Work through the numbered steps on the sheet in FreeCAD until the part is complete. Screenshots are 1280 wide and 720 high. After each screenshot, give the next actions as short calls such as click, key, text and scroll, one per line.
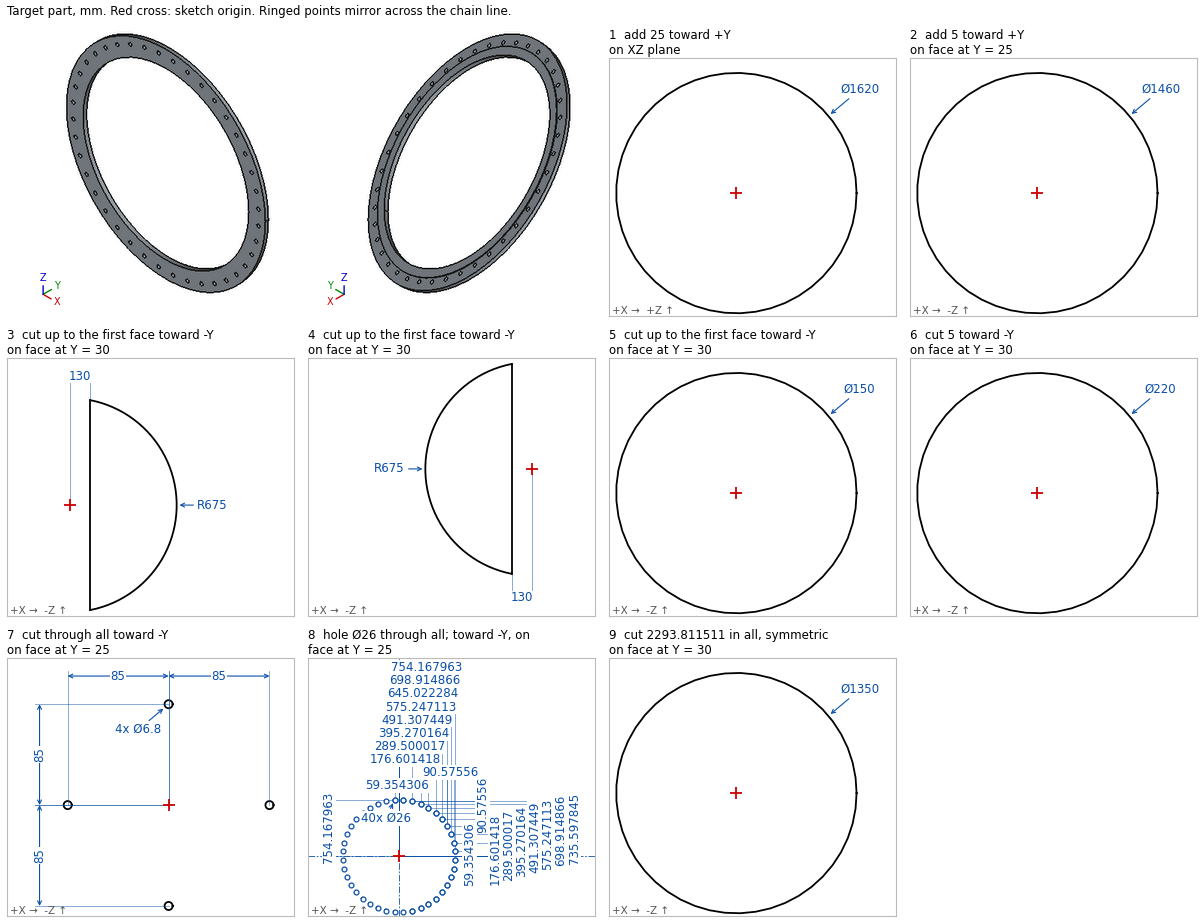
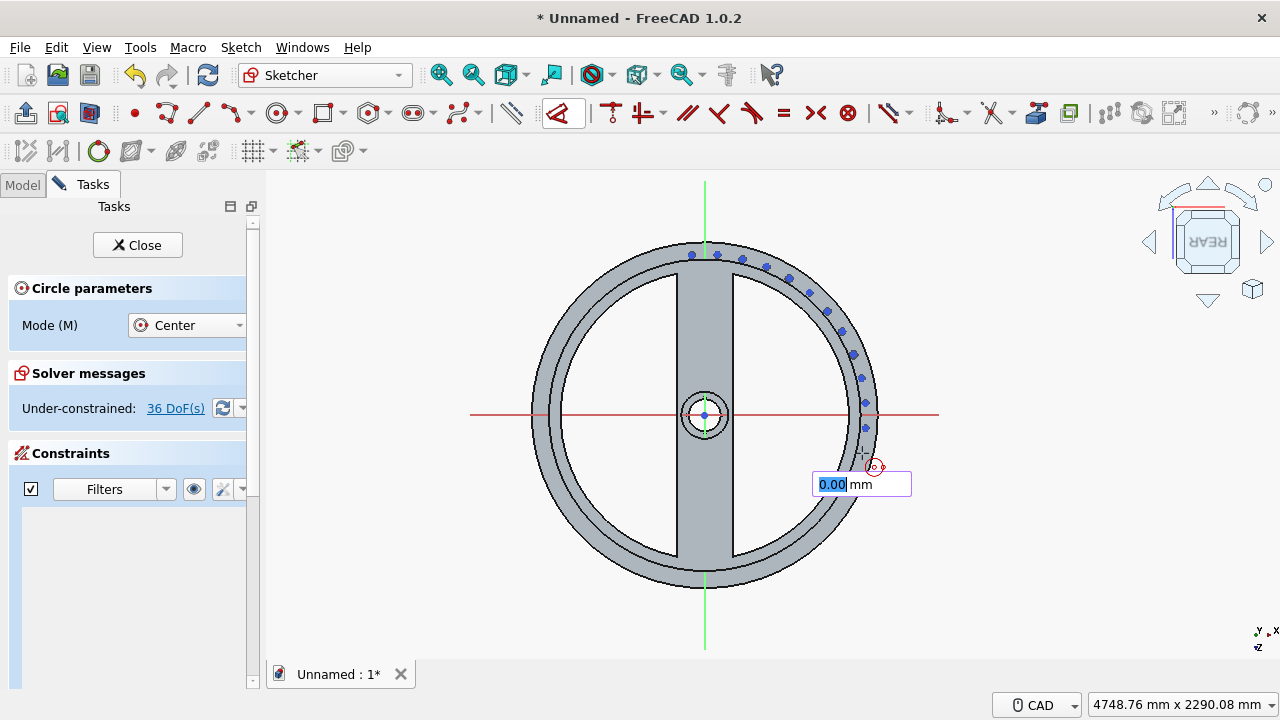
scroll(864, 451, up, 9)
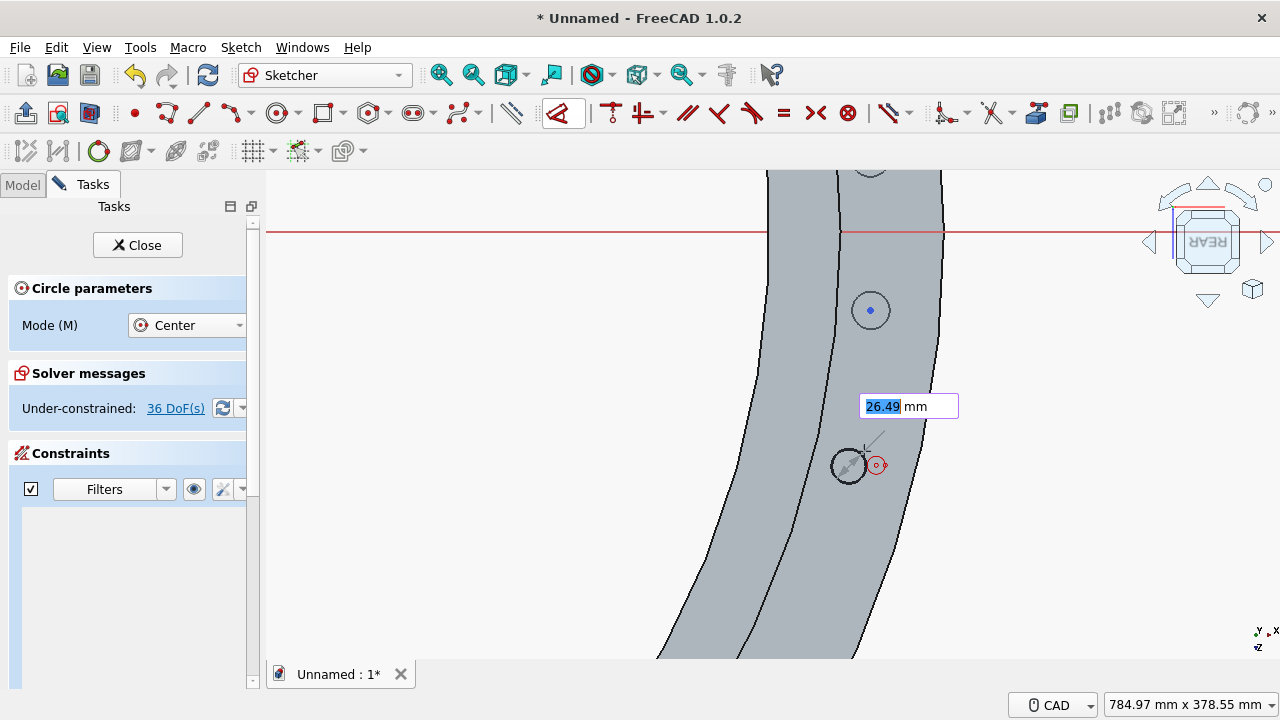
click(860, 448)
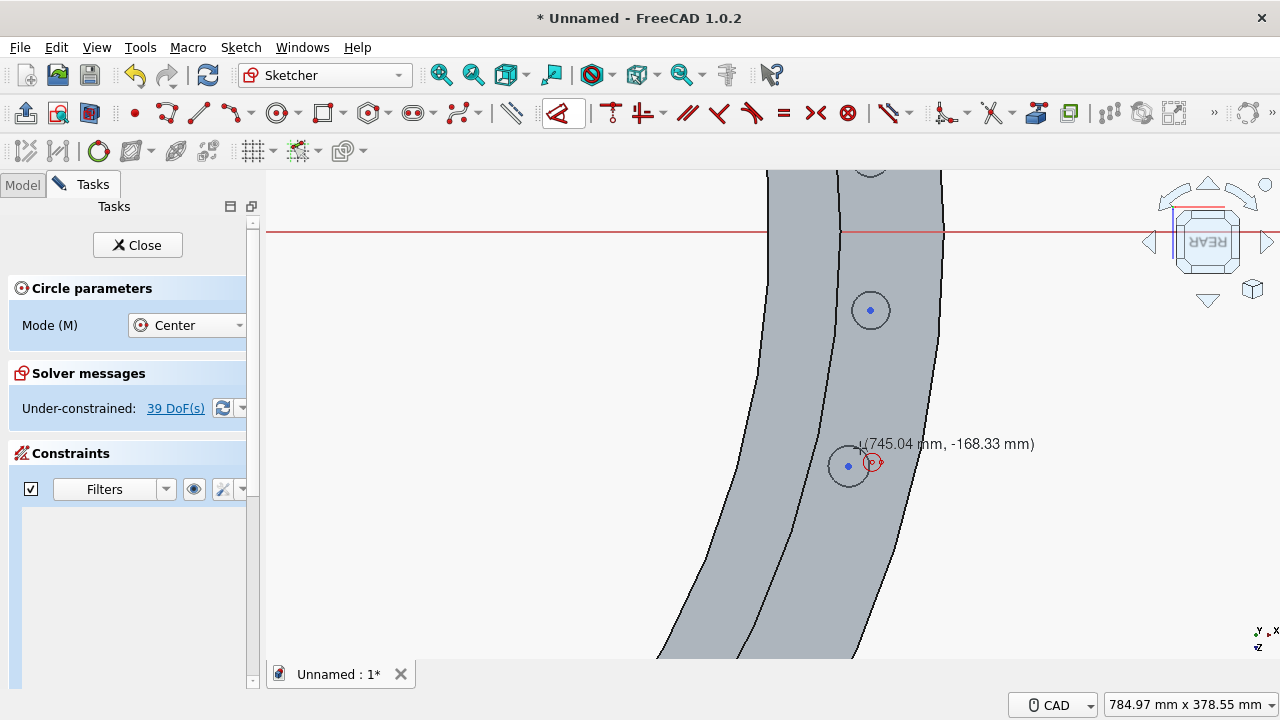
scroll(800, 606, up, 2)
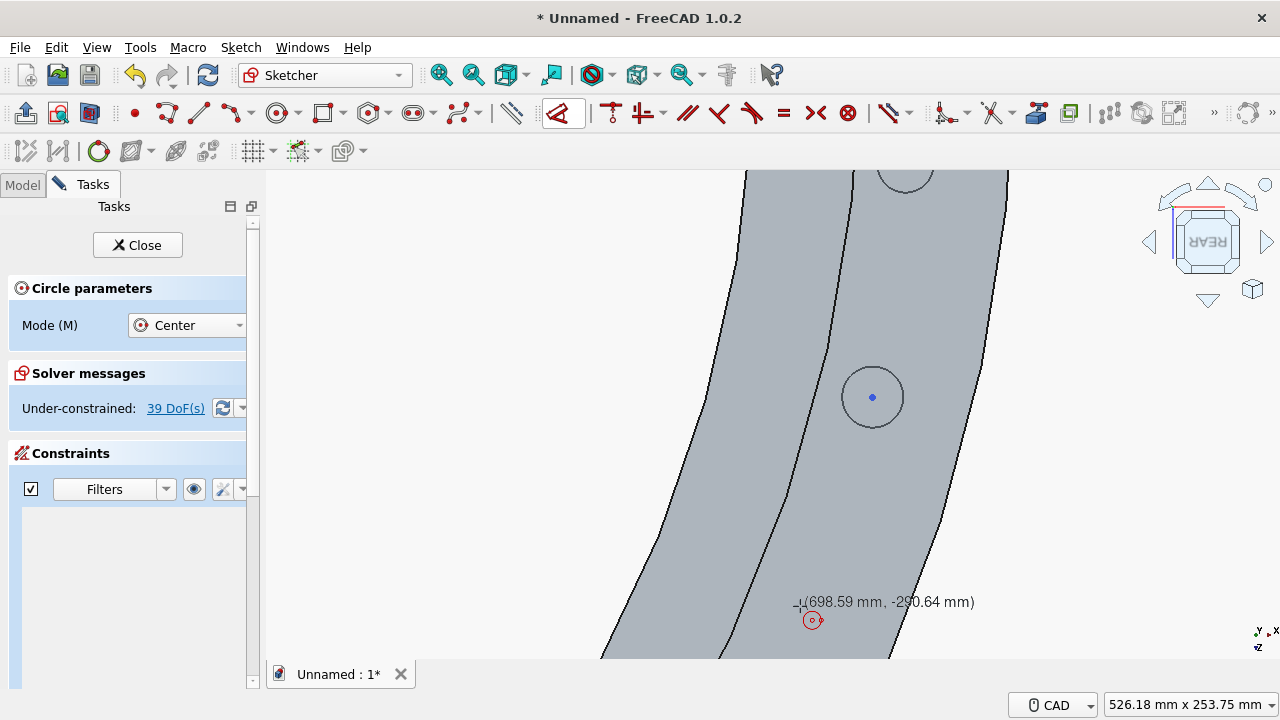
scroll(860, 460, down, 11)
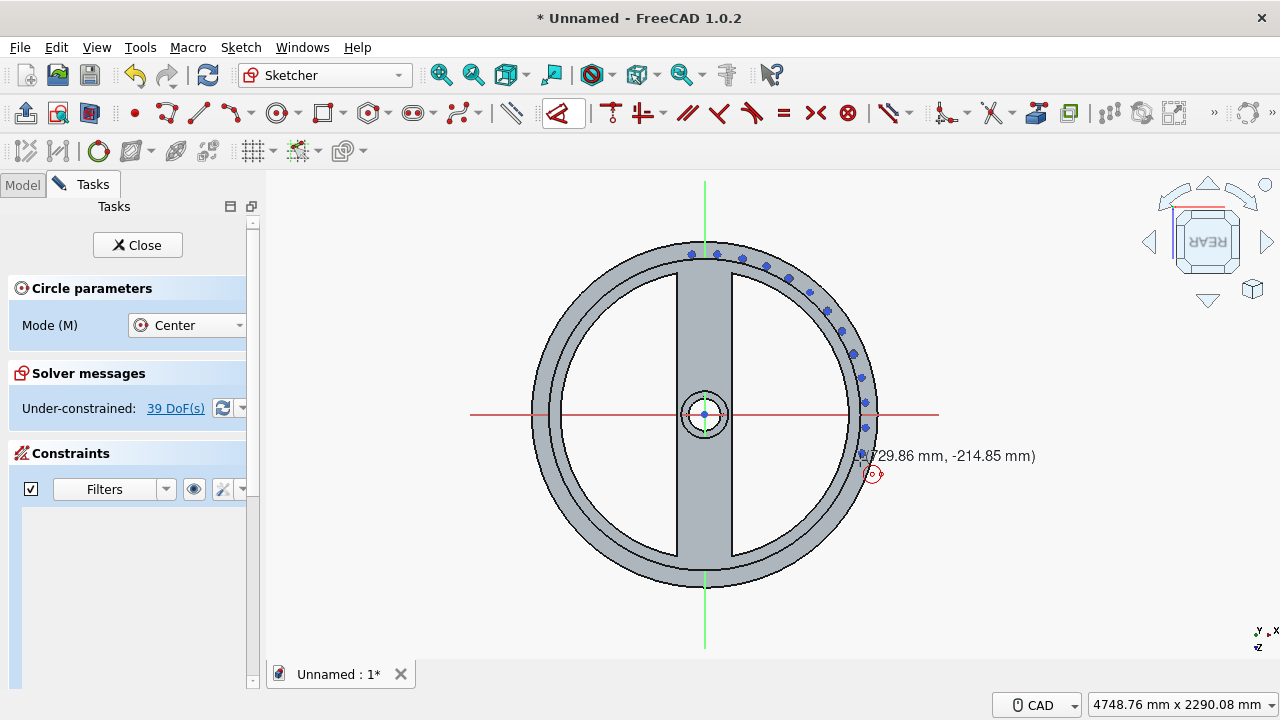
click(854, 477)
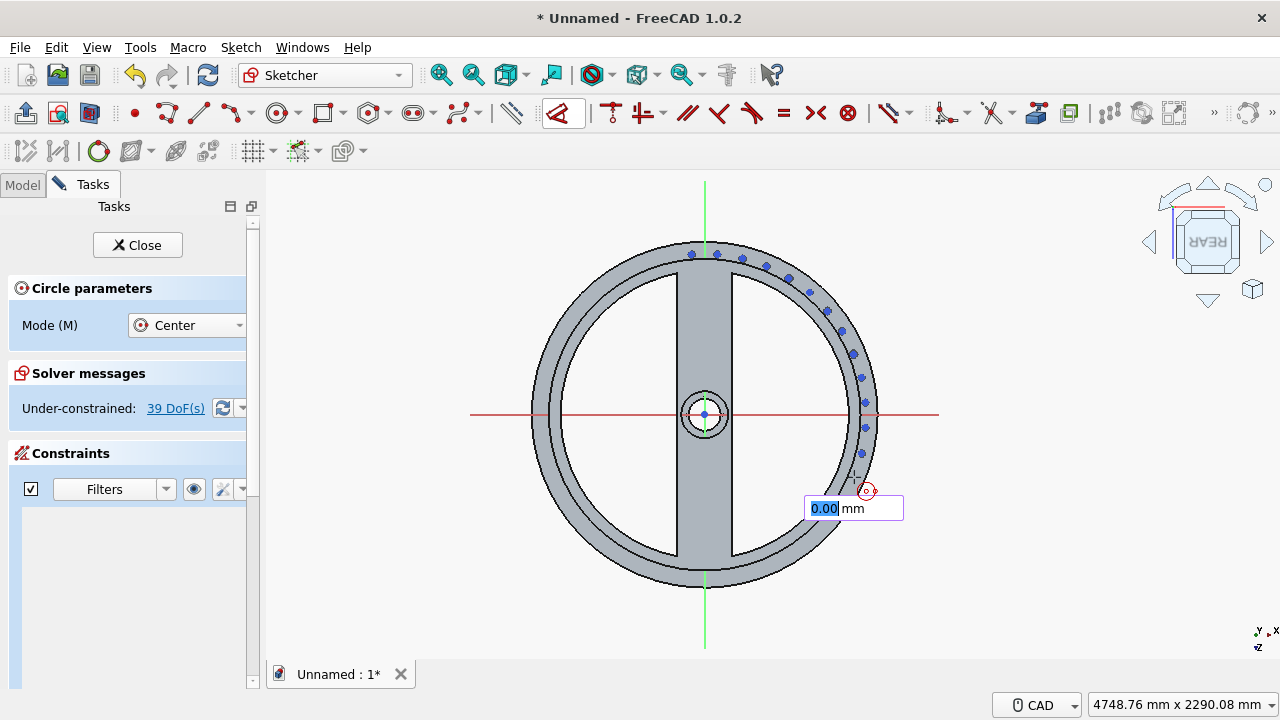
scroll(856, 475, up, 9)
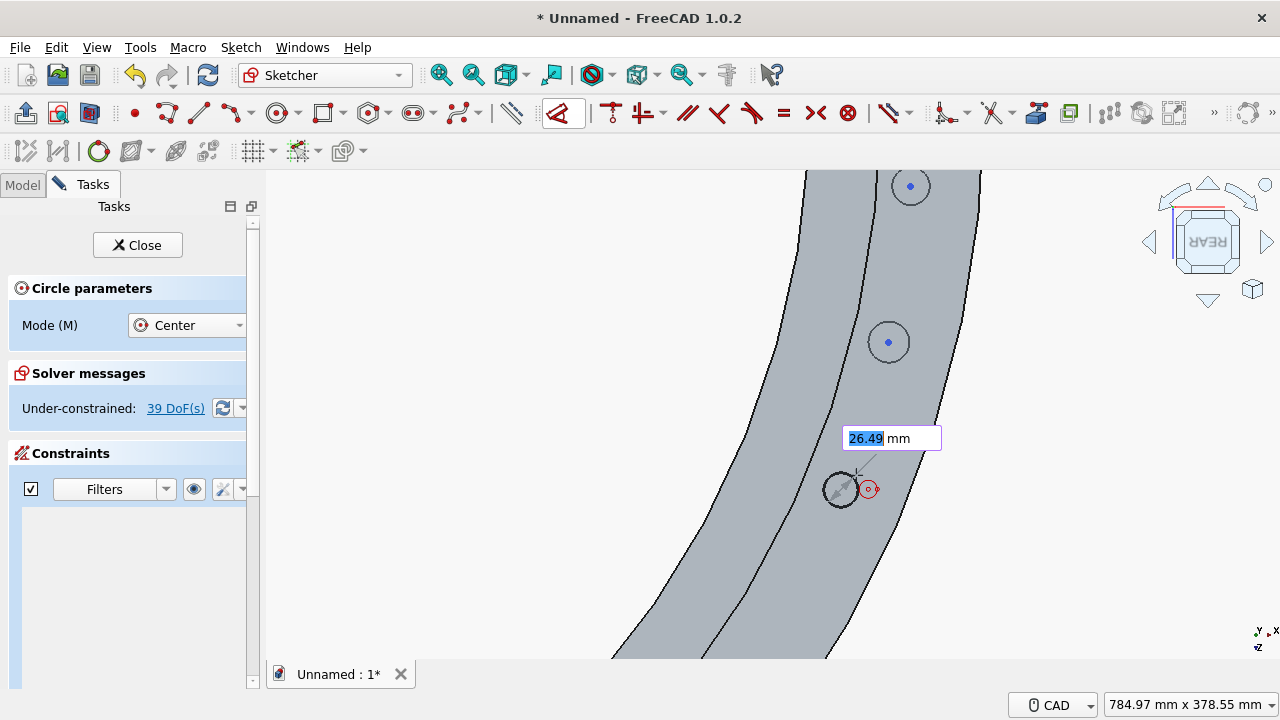
click(852, 470)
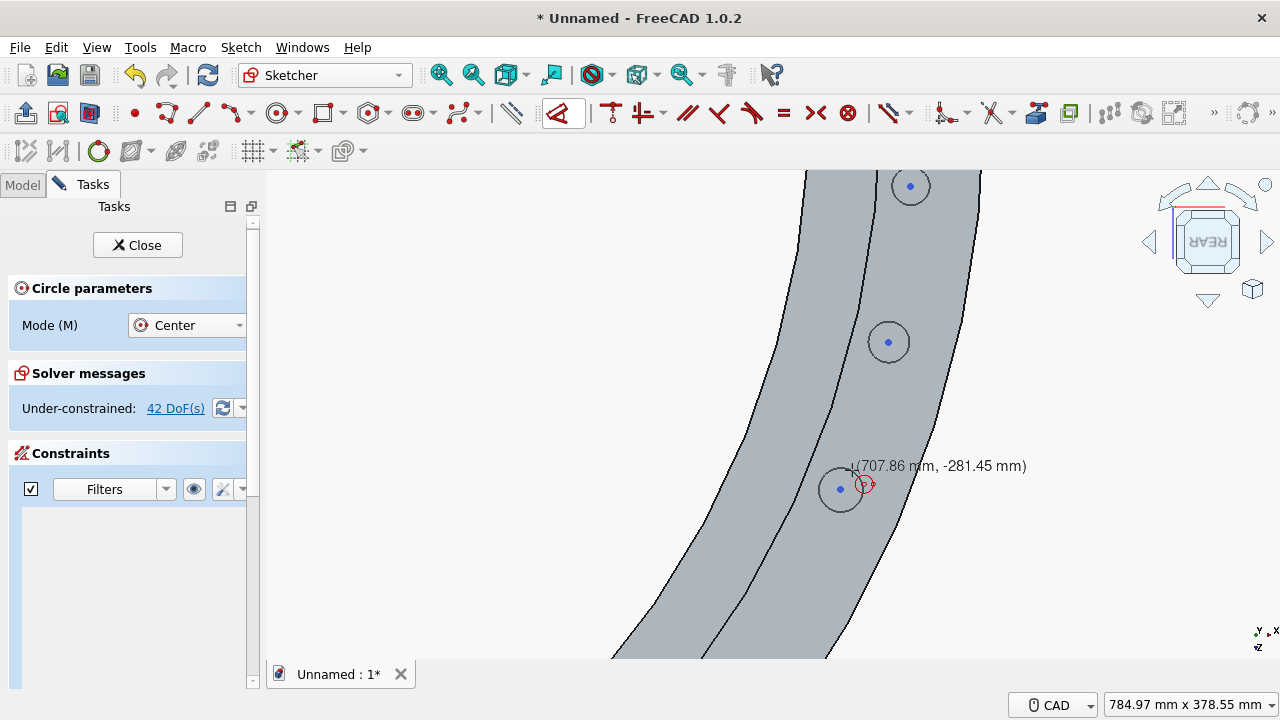
scroll(771, 618, up, 2)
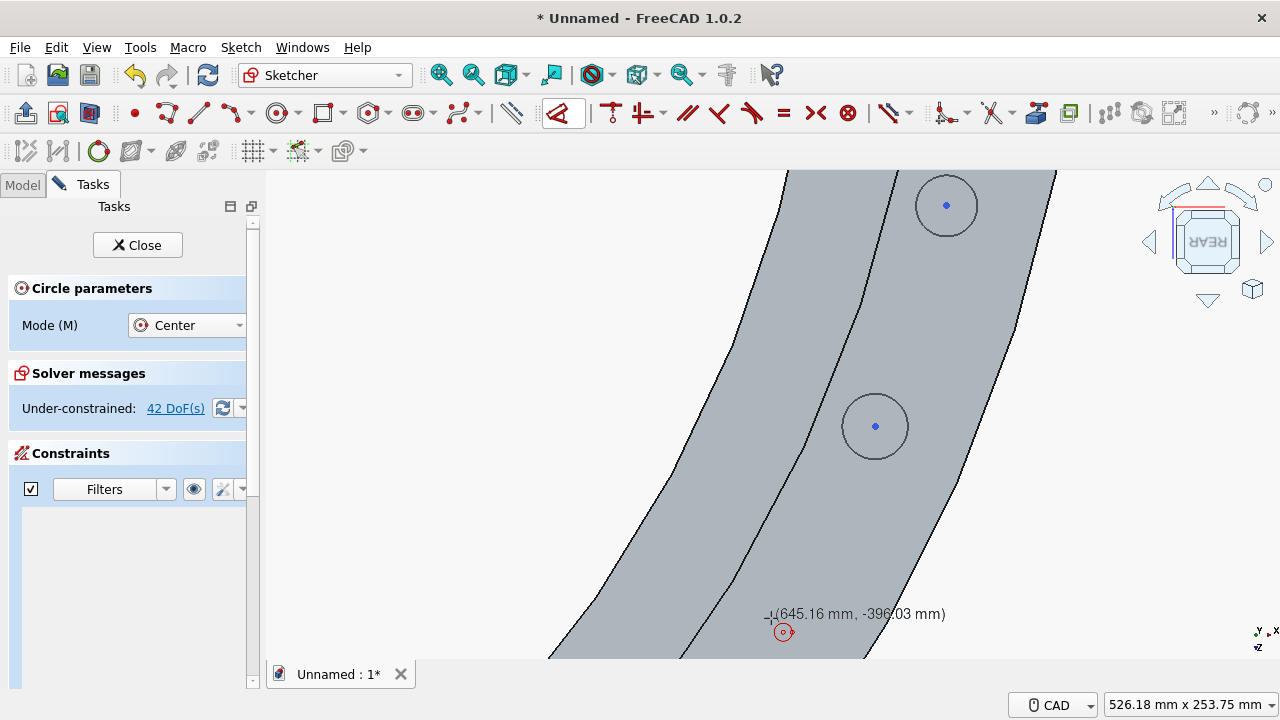
scroll(851, 484, down, 11)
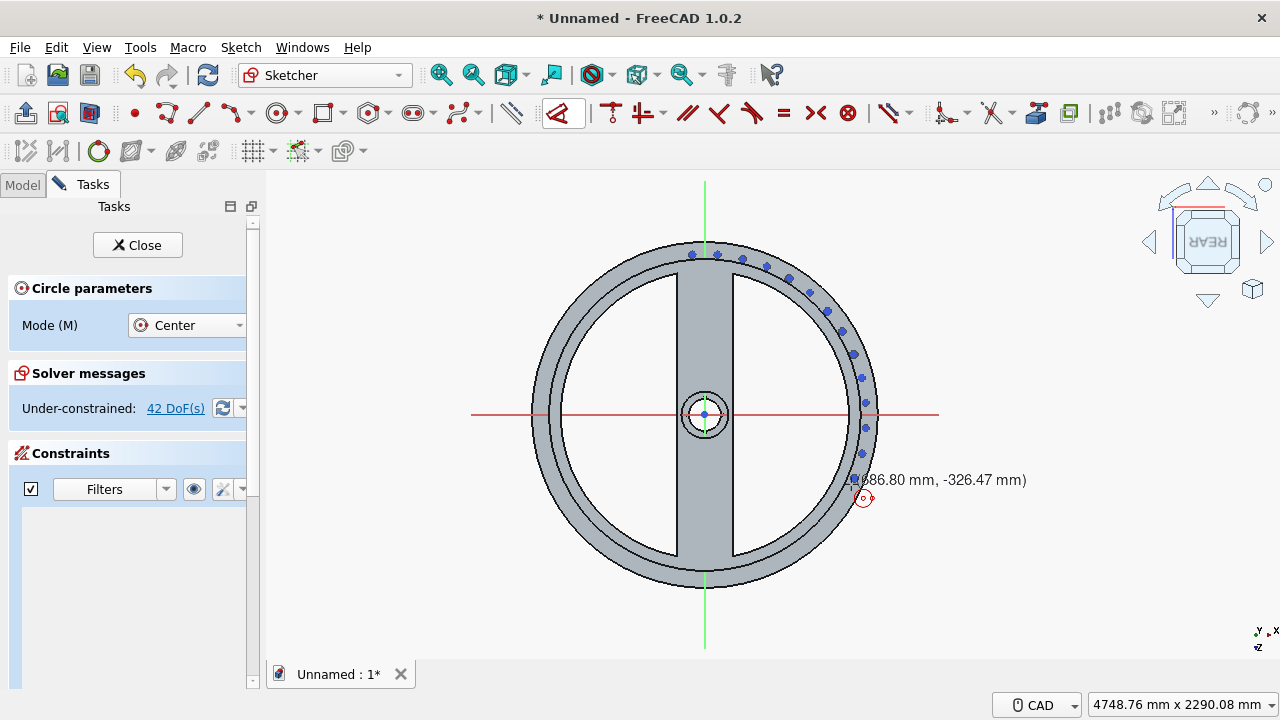
click(843, 499)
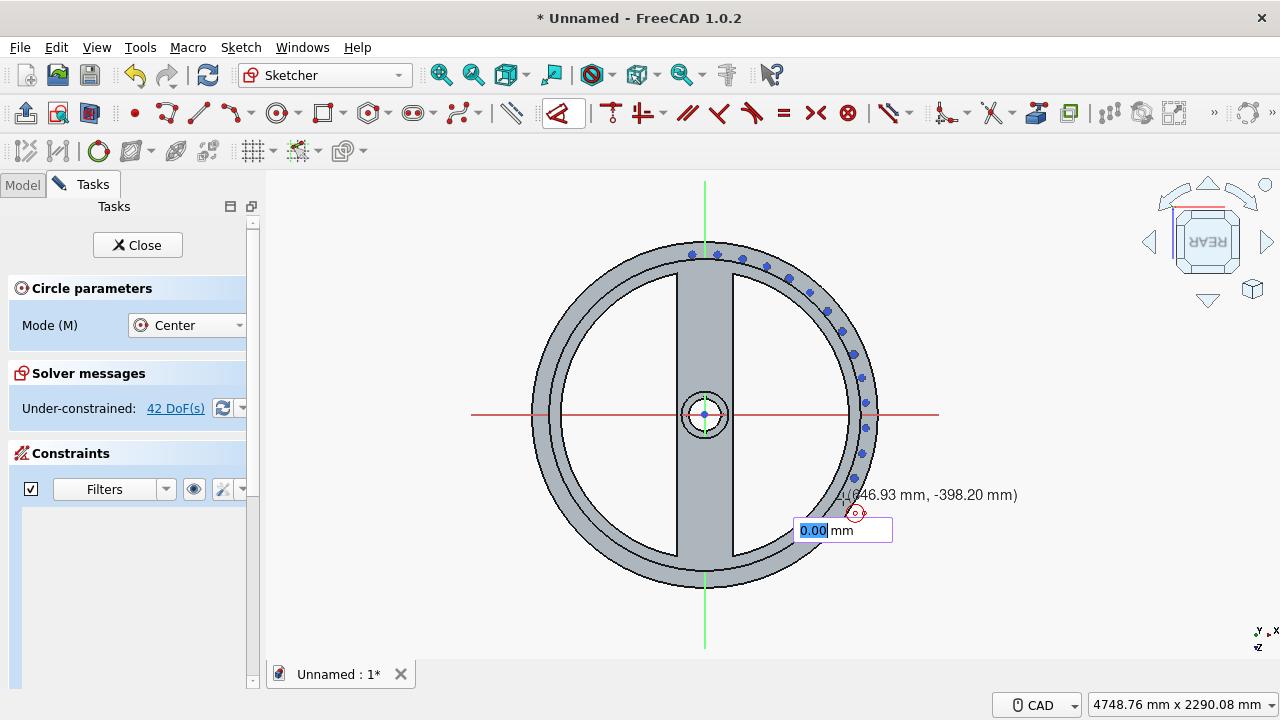
scroll(845, 497, up, 9)